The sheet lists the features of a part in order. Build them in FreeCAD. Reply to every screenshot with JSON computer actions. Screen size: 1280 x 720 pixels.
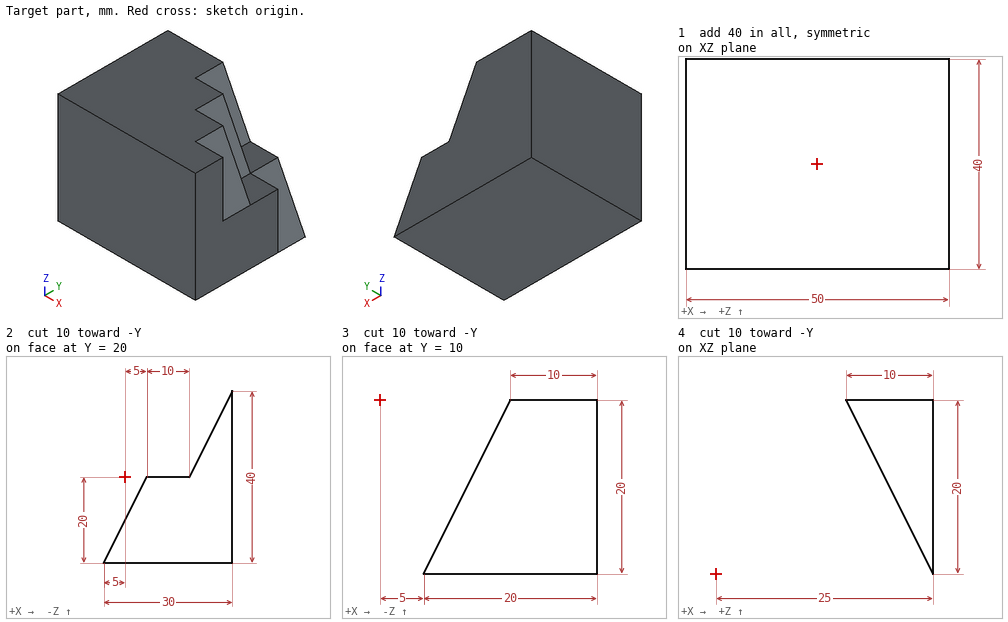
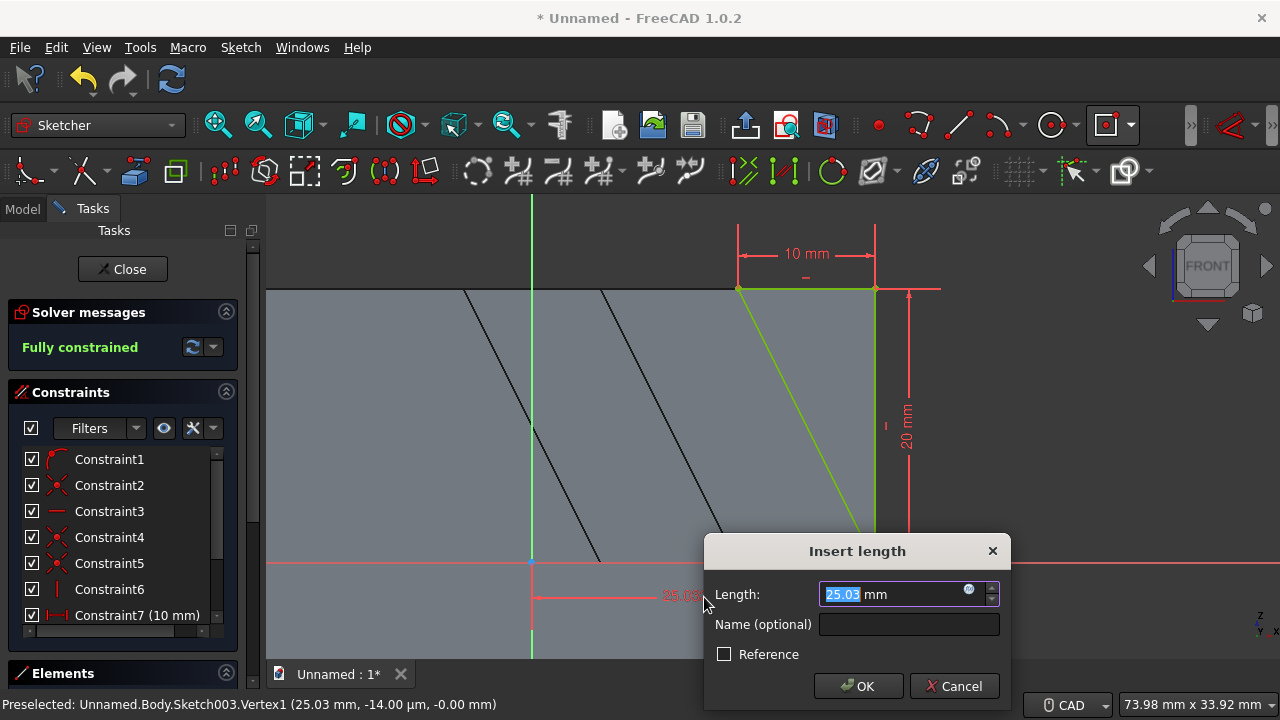
{"action": "type", "text": "25"}
{"action": "key", "text": "Return"}
{"action": "key", "text": "Escape"}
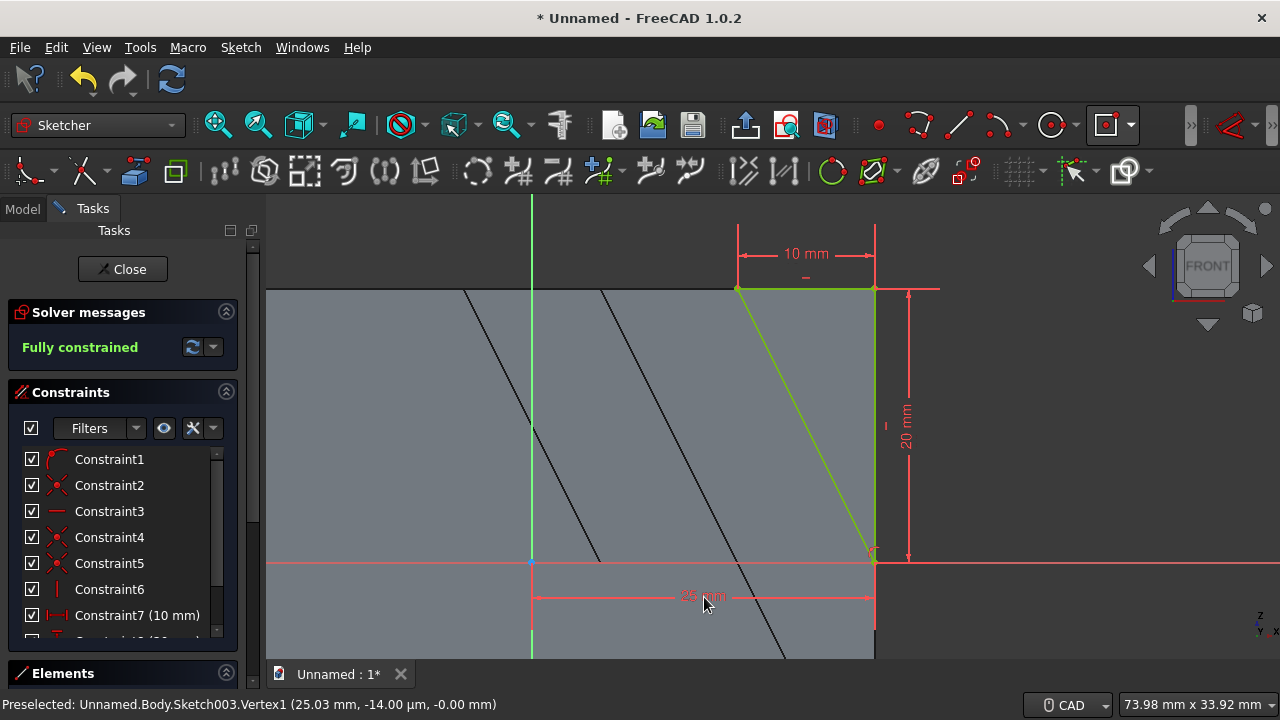
{"action": "left_click", "coordinate": [123, 269]}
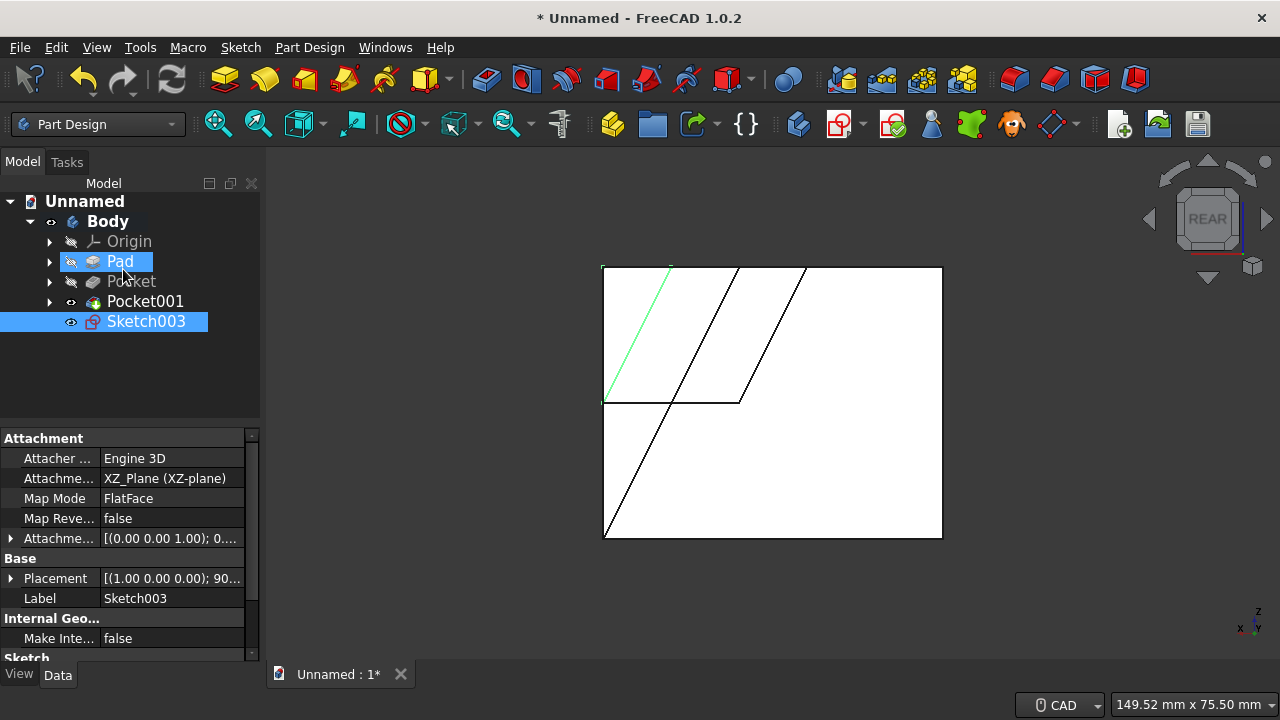
{"action": "left_click", "coordinate": [488, 80]}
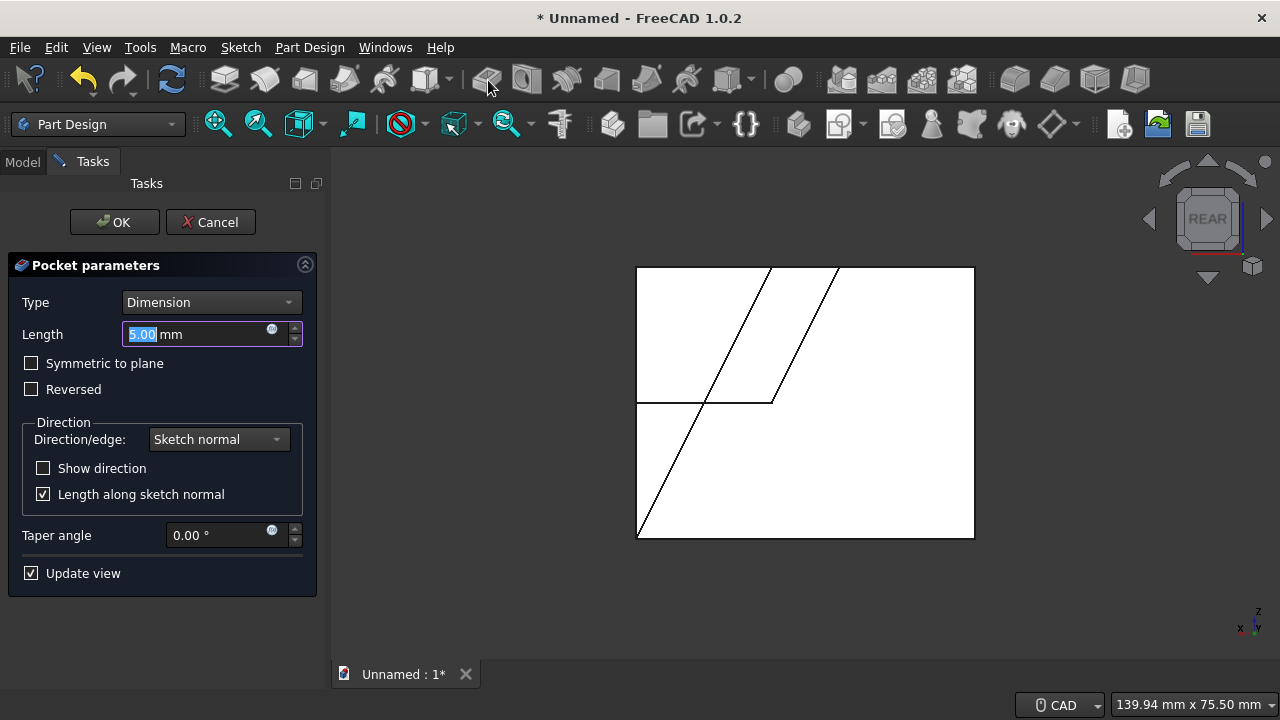
{"action": "type", "text": "10"}
{"action": "key", "text": "Tab"}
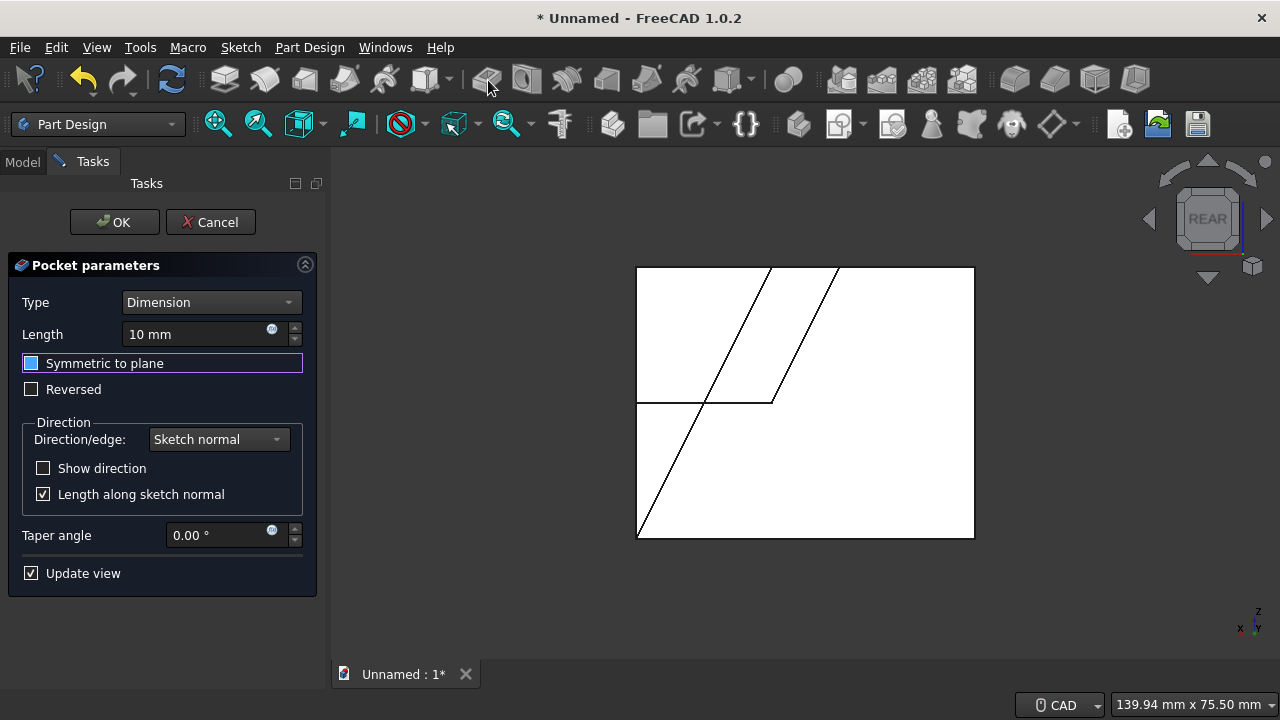
{"action": "left_click", "coordinate": [30, 389]}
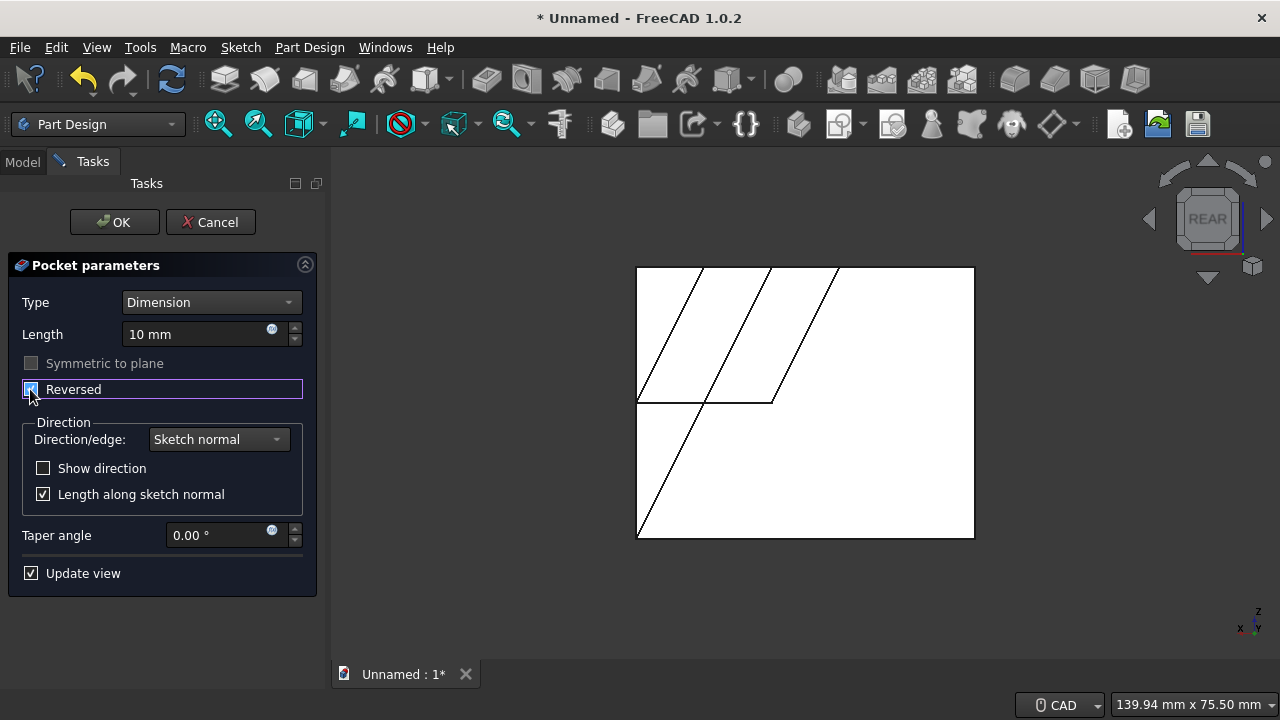
{"action": "left_click", "coordinate": [115, 222]}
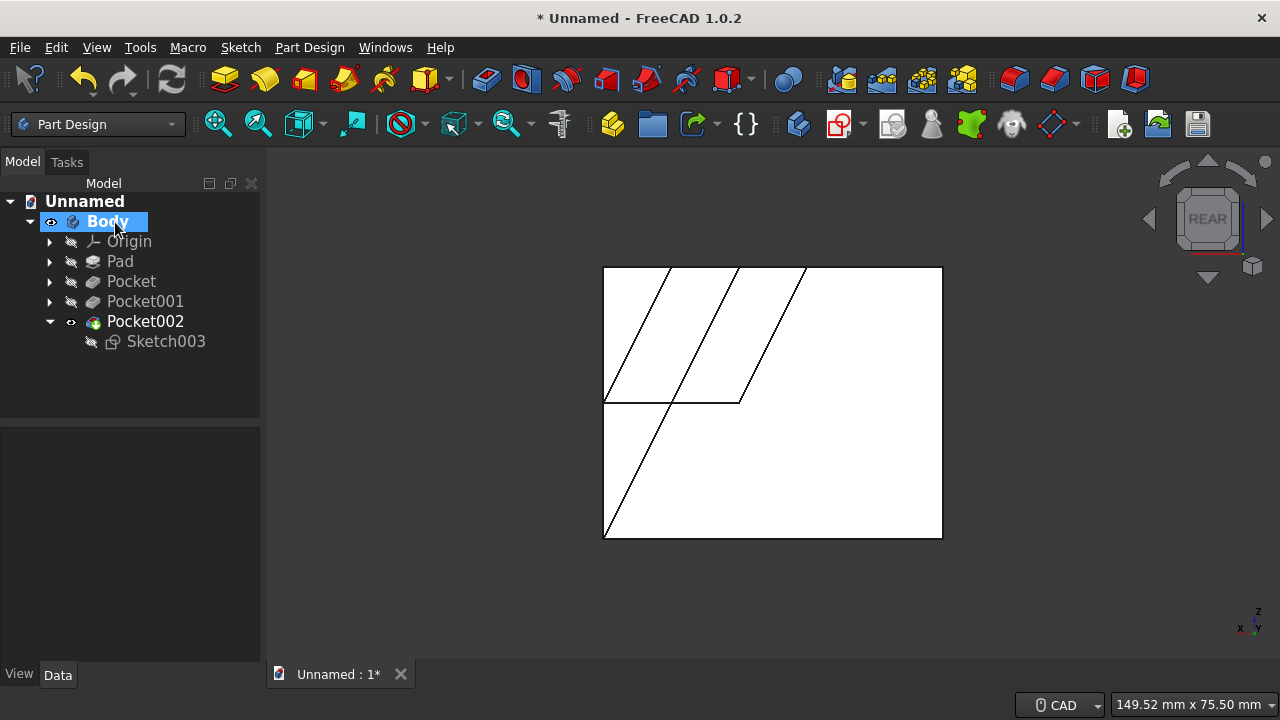
{"action": "key", "text": "0"}